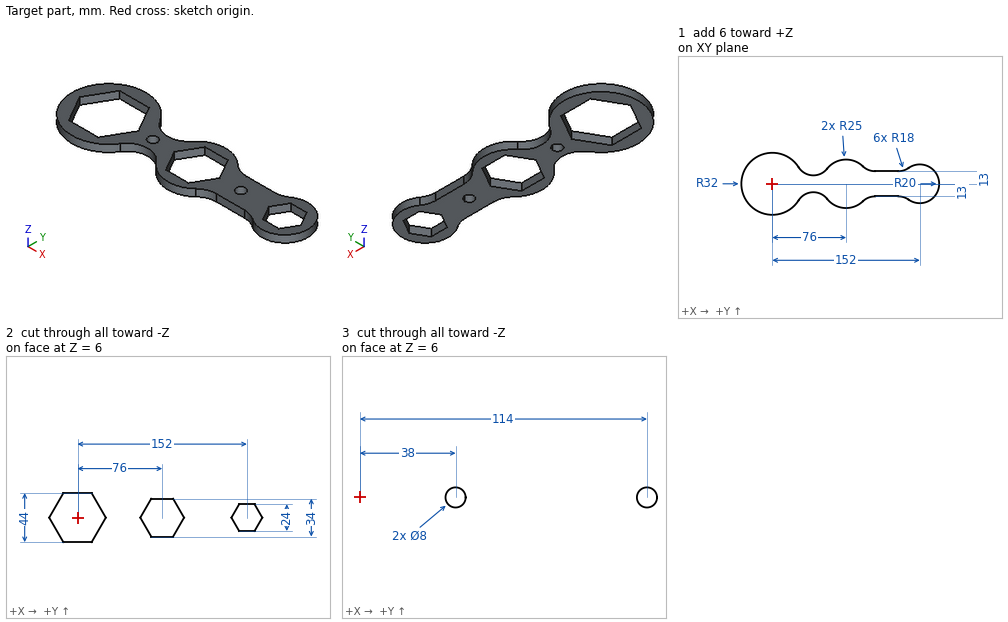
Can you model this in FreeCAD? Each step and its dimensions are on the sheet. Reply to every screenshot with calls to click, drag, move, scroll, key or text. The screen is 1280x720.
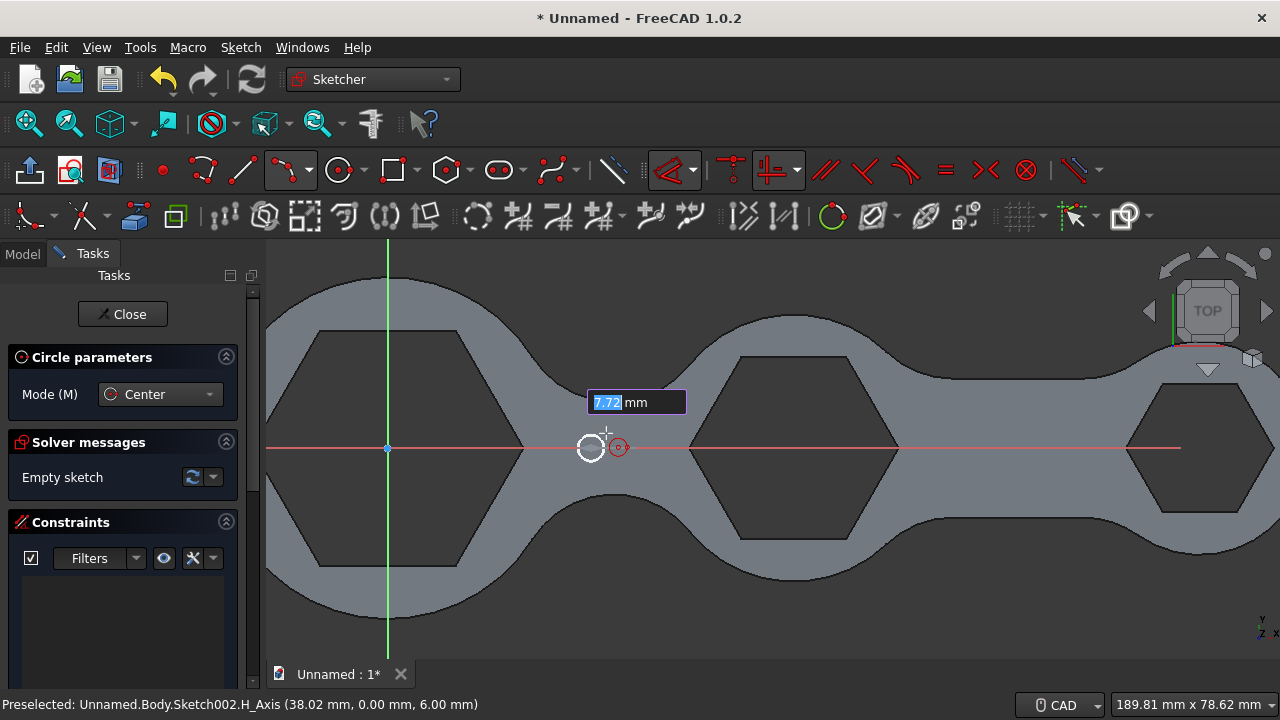
text(8)
key(Return)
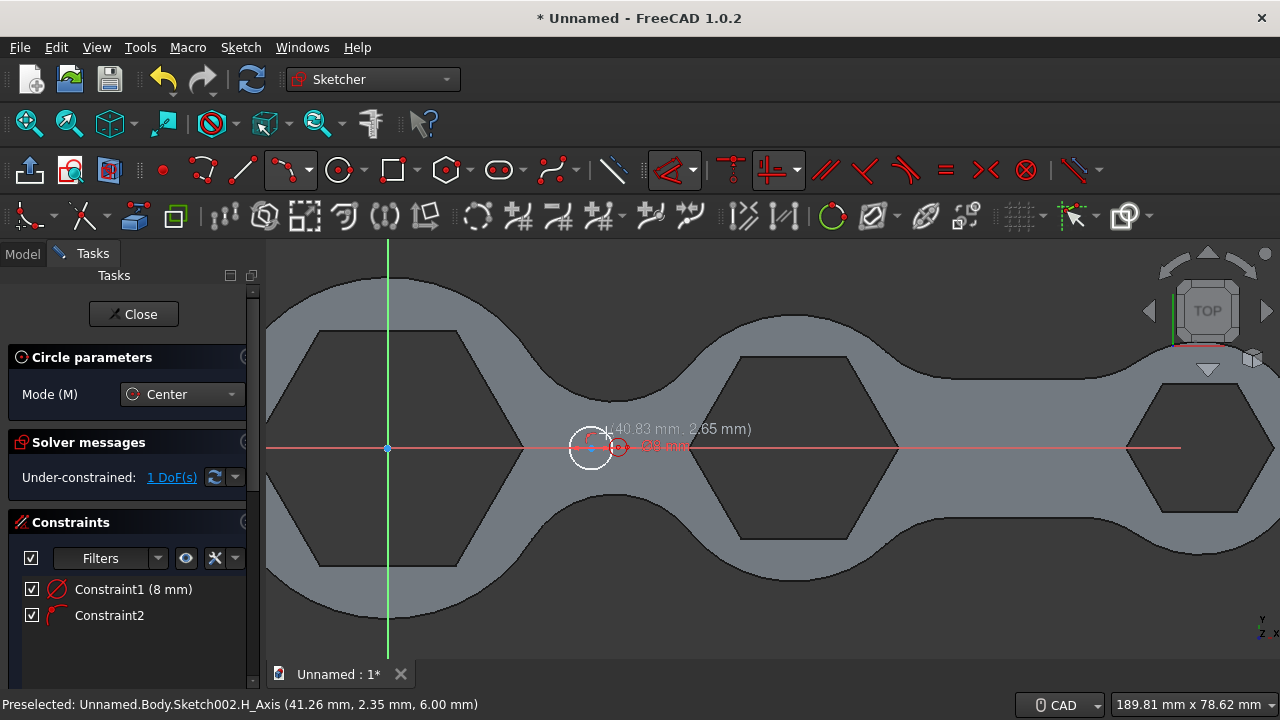
click(997, 448)
move(1012, 433)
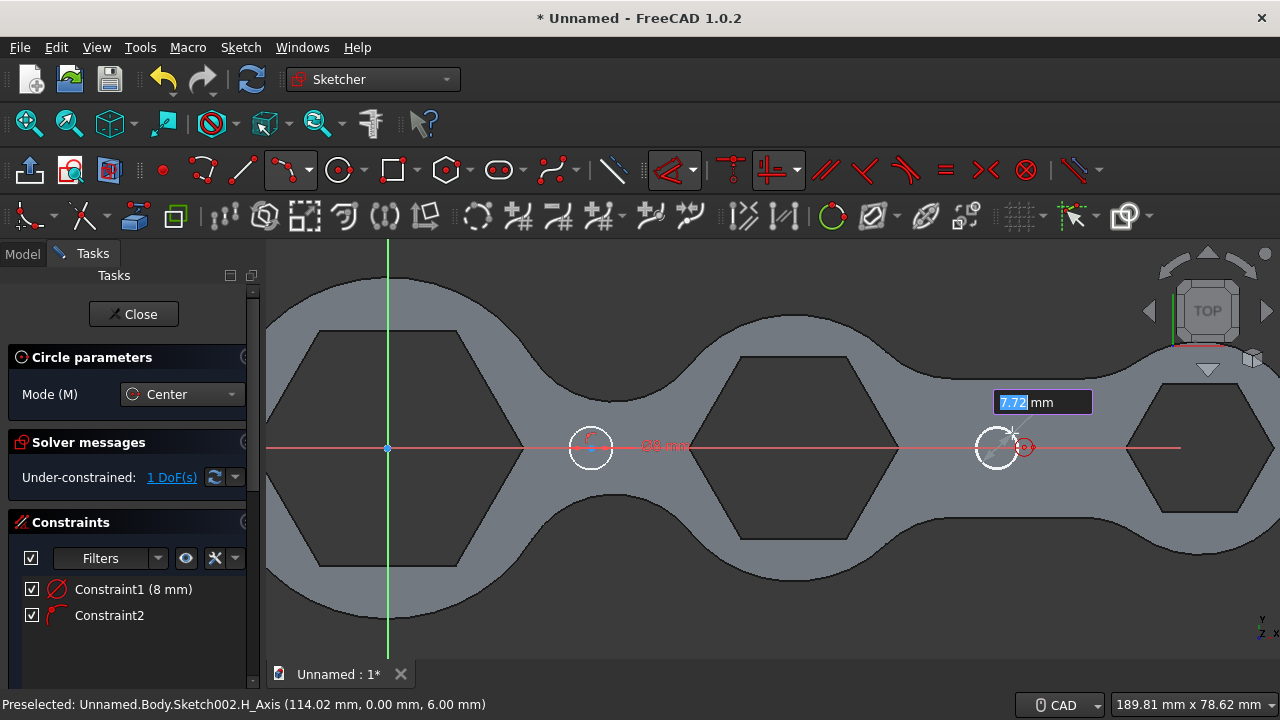
text(8)
key(Return)
key(Escape)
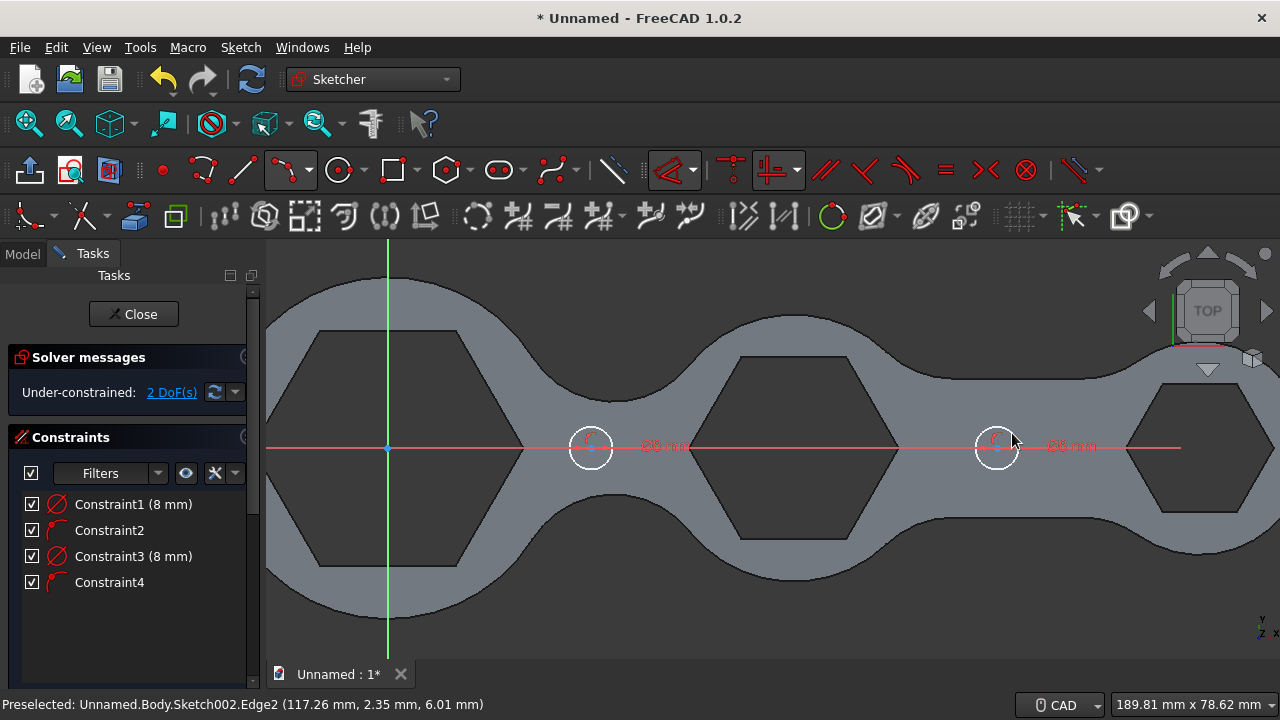
click(591, 448)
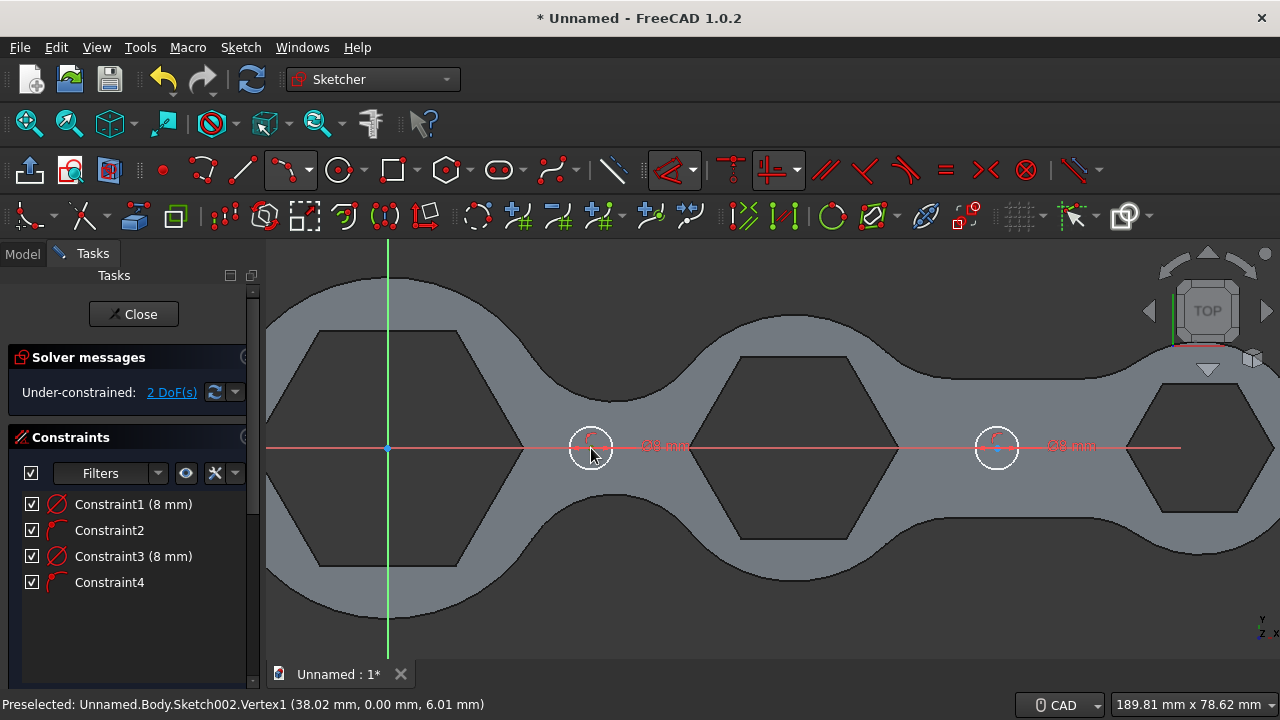
key(l)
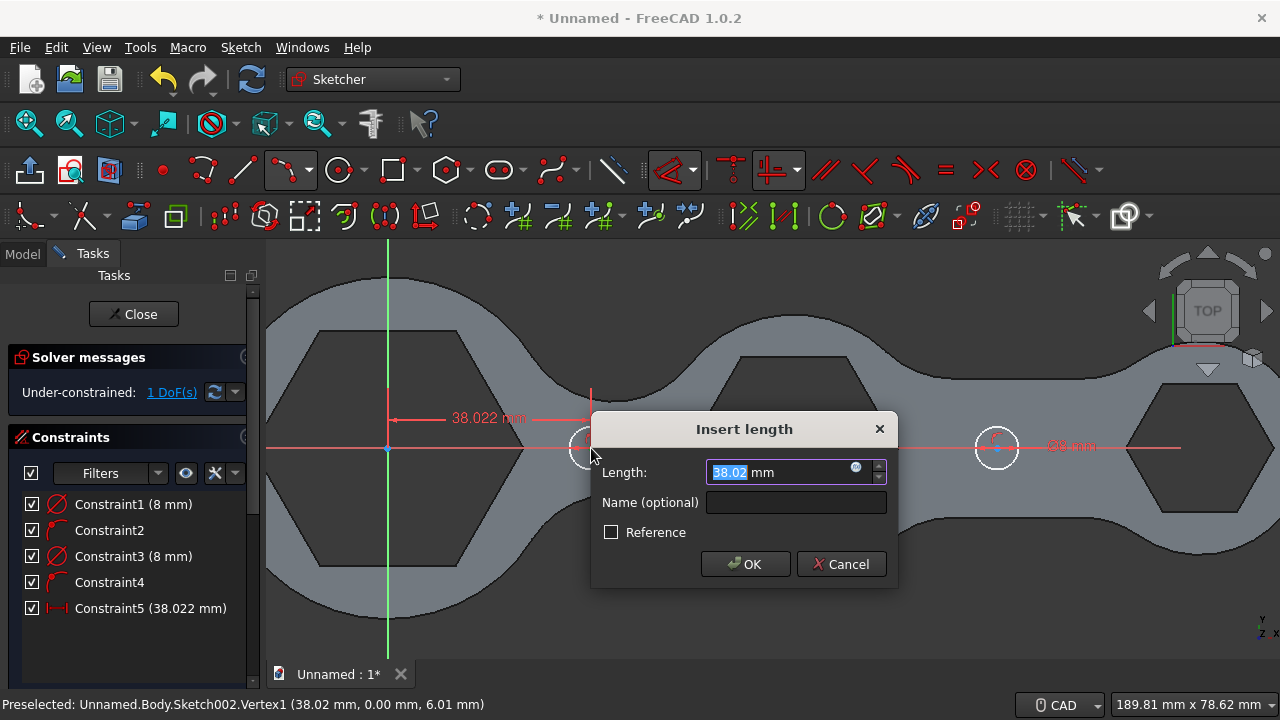
text(38)
key(Return)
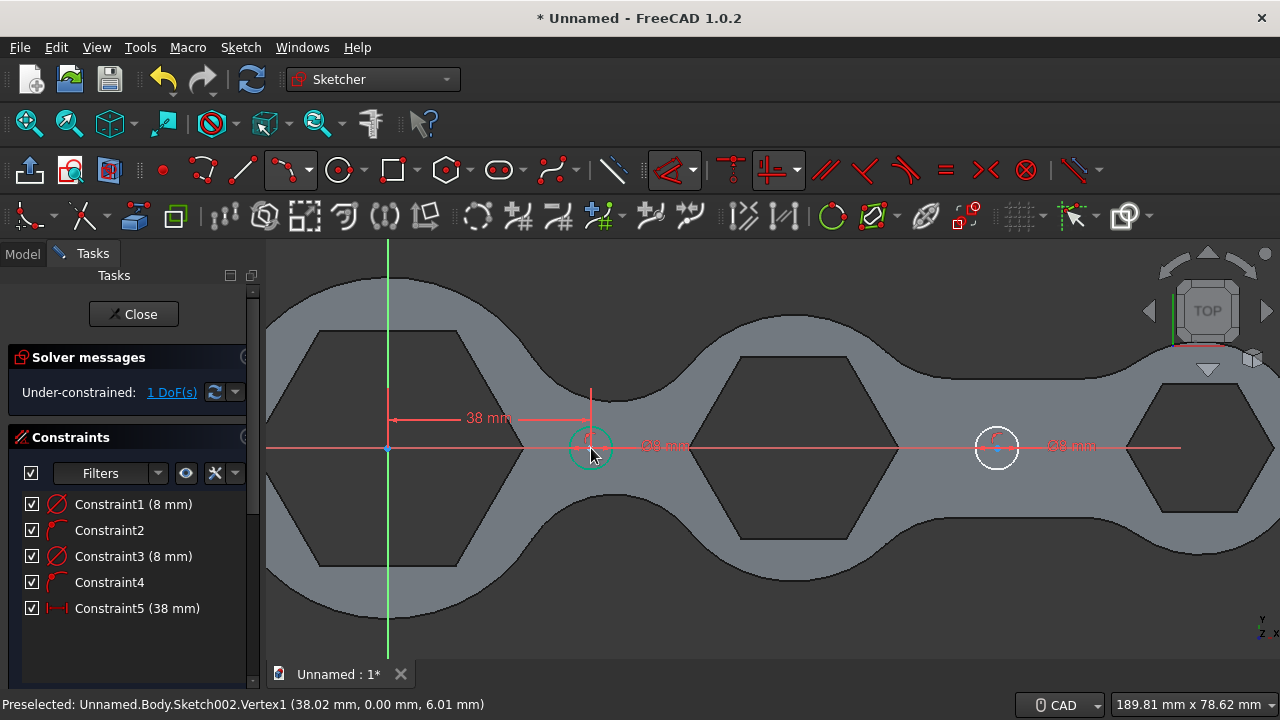
click(997, 448)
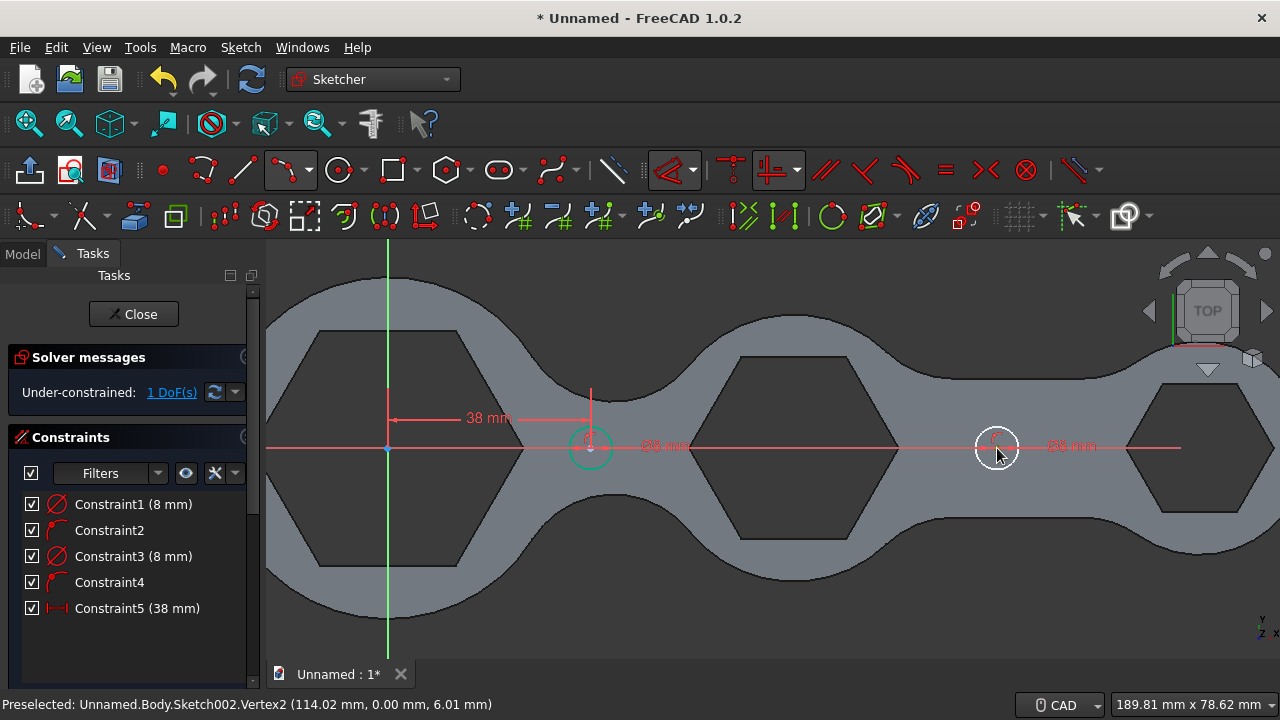
click(696, 170)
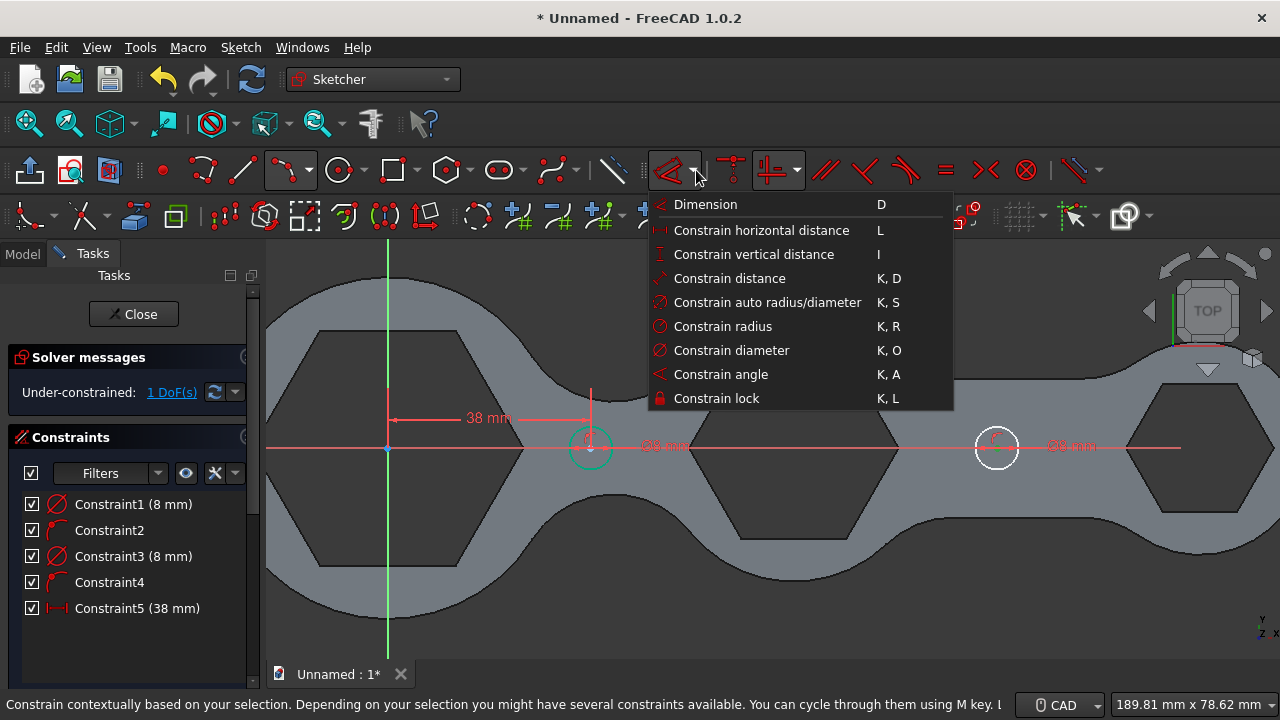
click(801, 230)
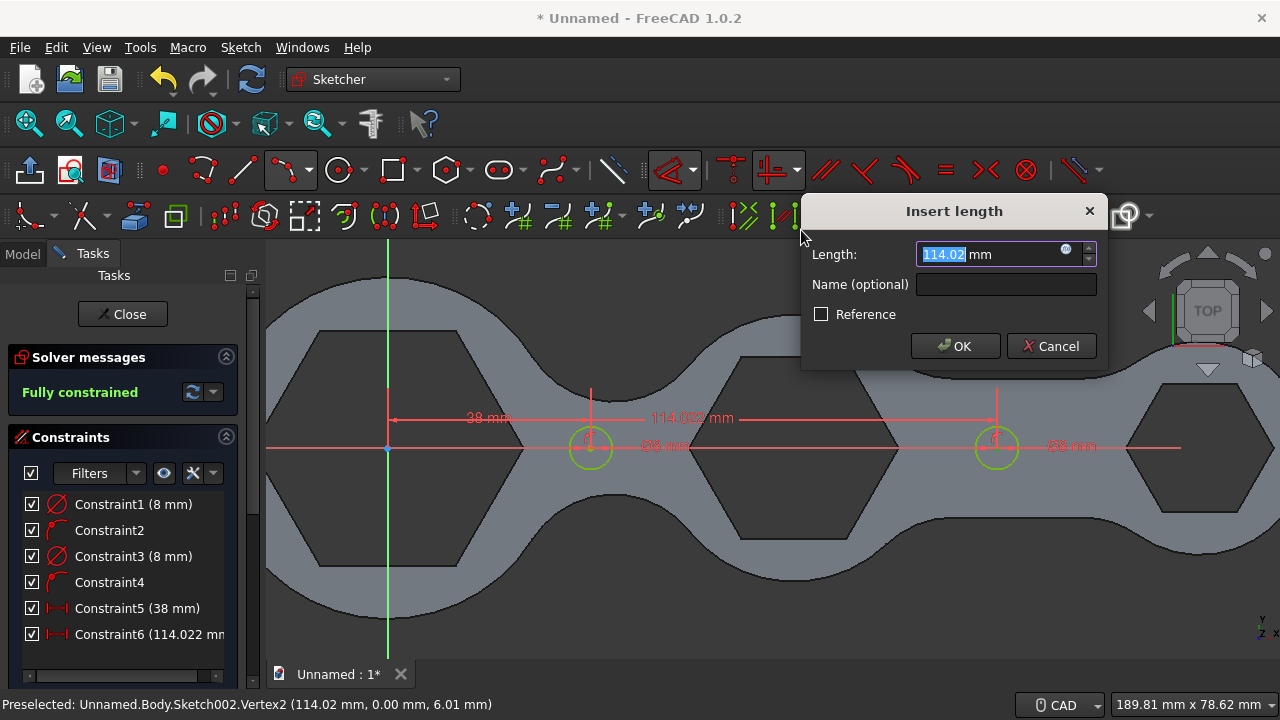
text(114)
key(Return)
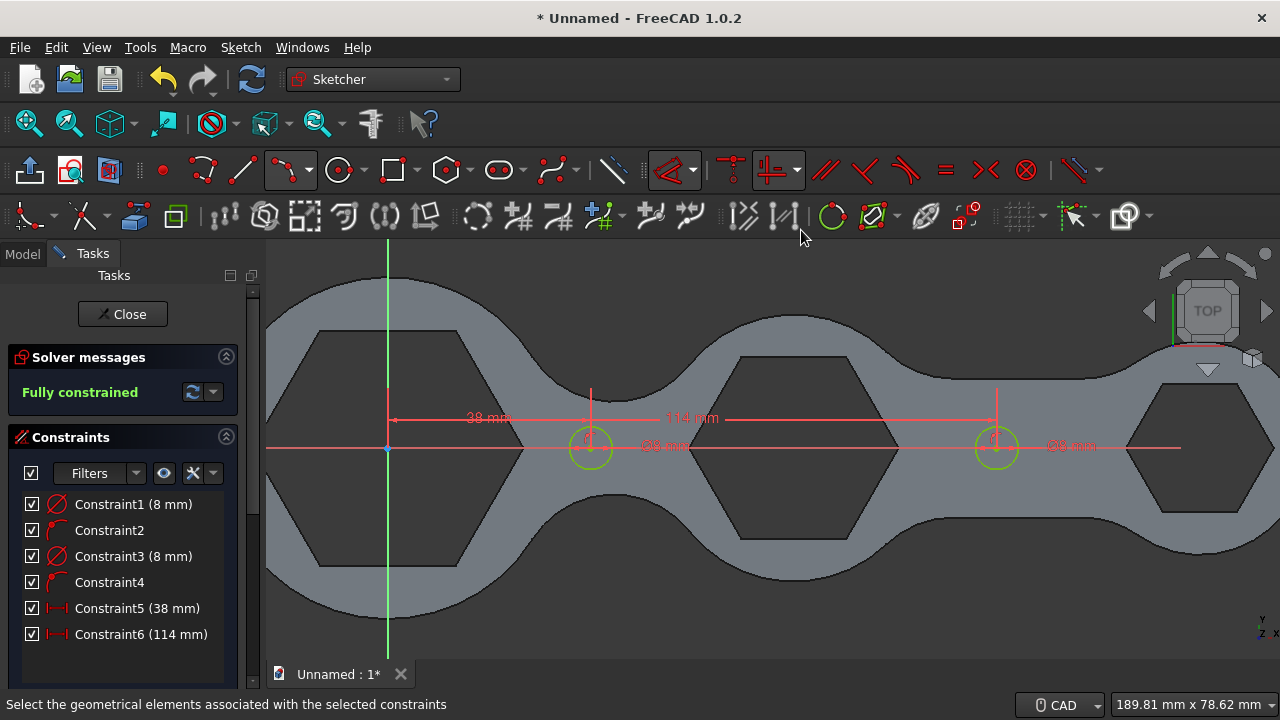
click(123, 314)